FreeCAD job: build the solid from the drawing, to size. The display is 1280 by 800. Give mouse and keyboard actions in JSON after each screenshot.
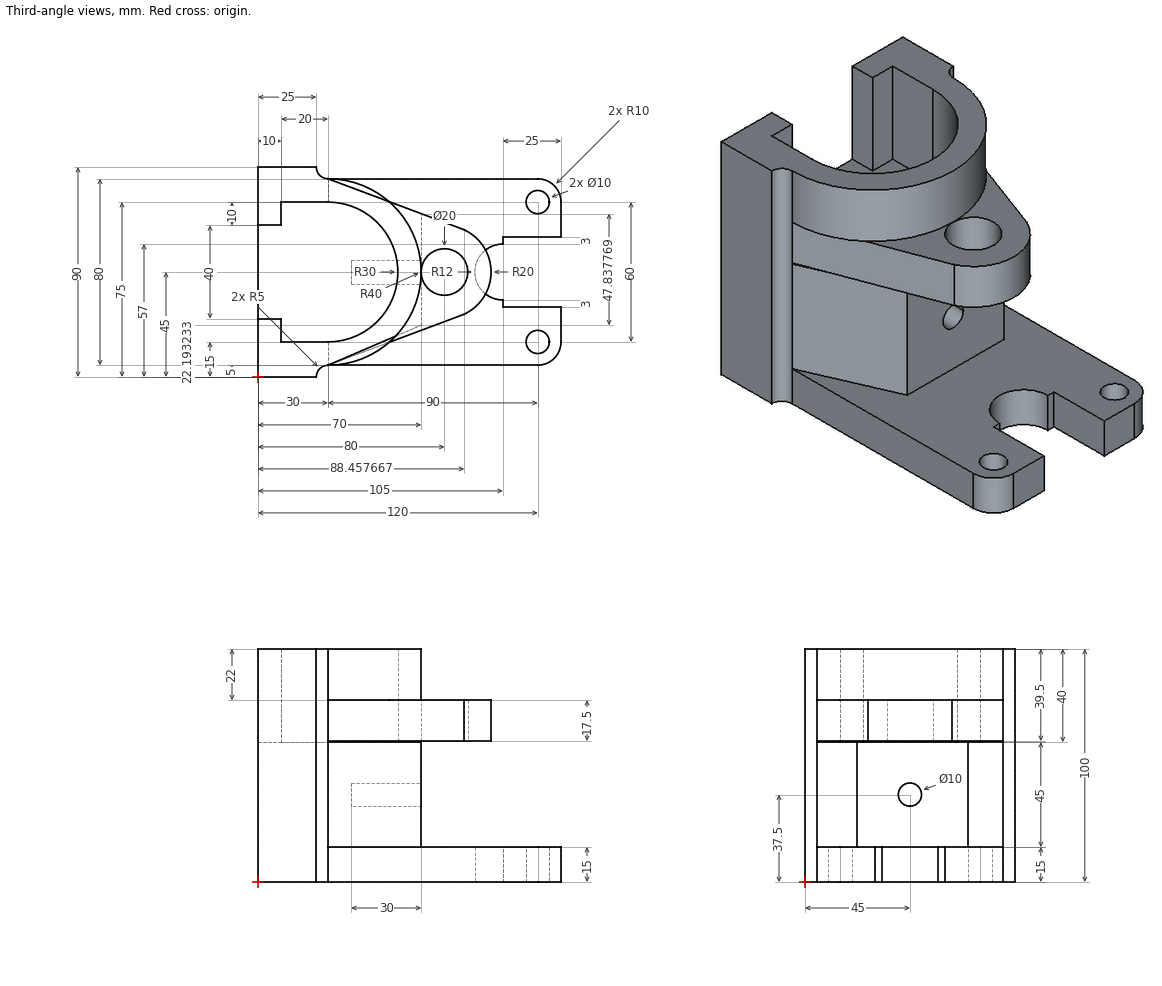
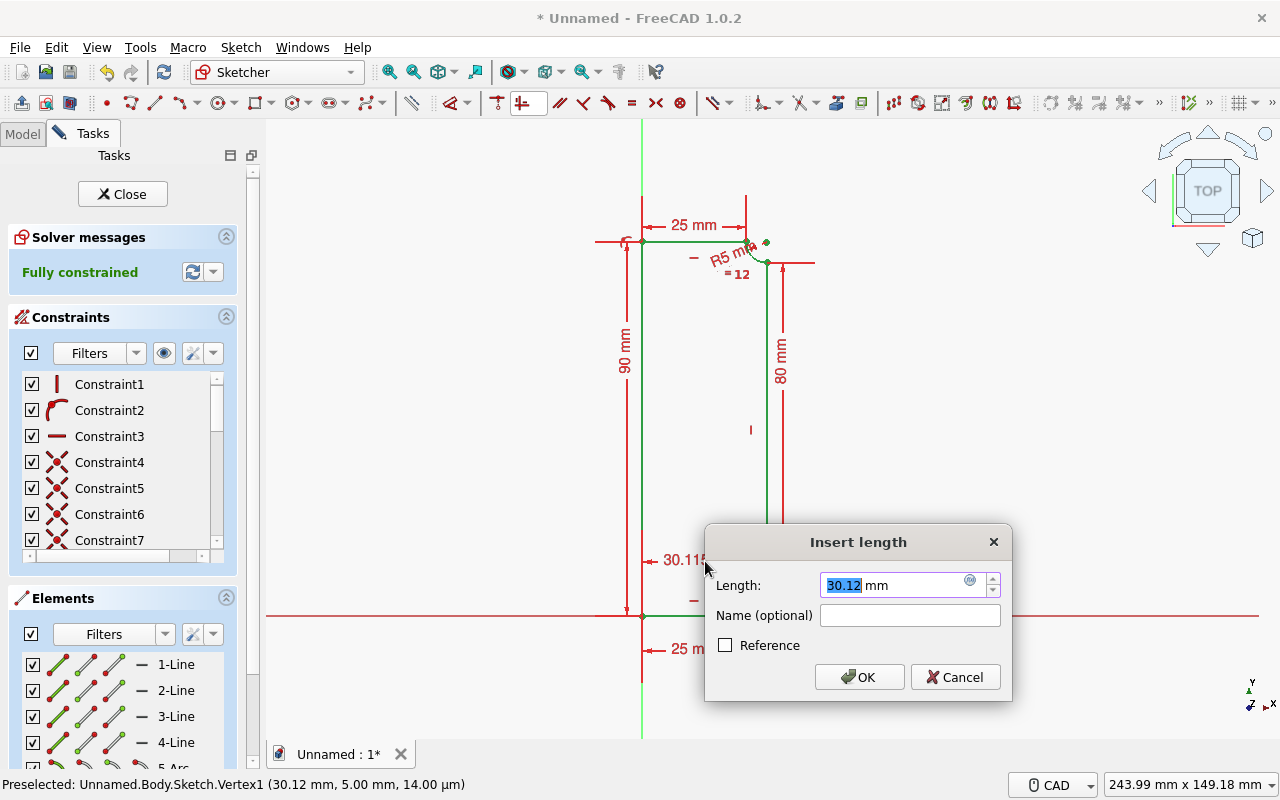
{"action": "type", "text": "30"}
{"action": "key", "text": "Return"}
{"action": "key", "text": "Escape"}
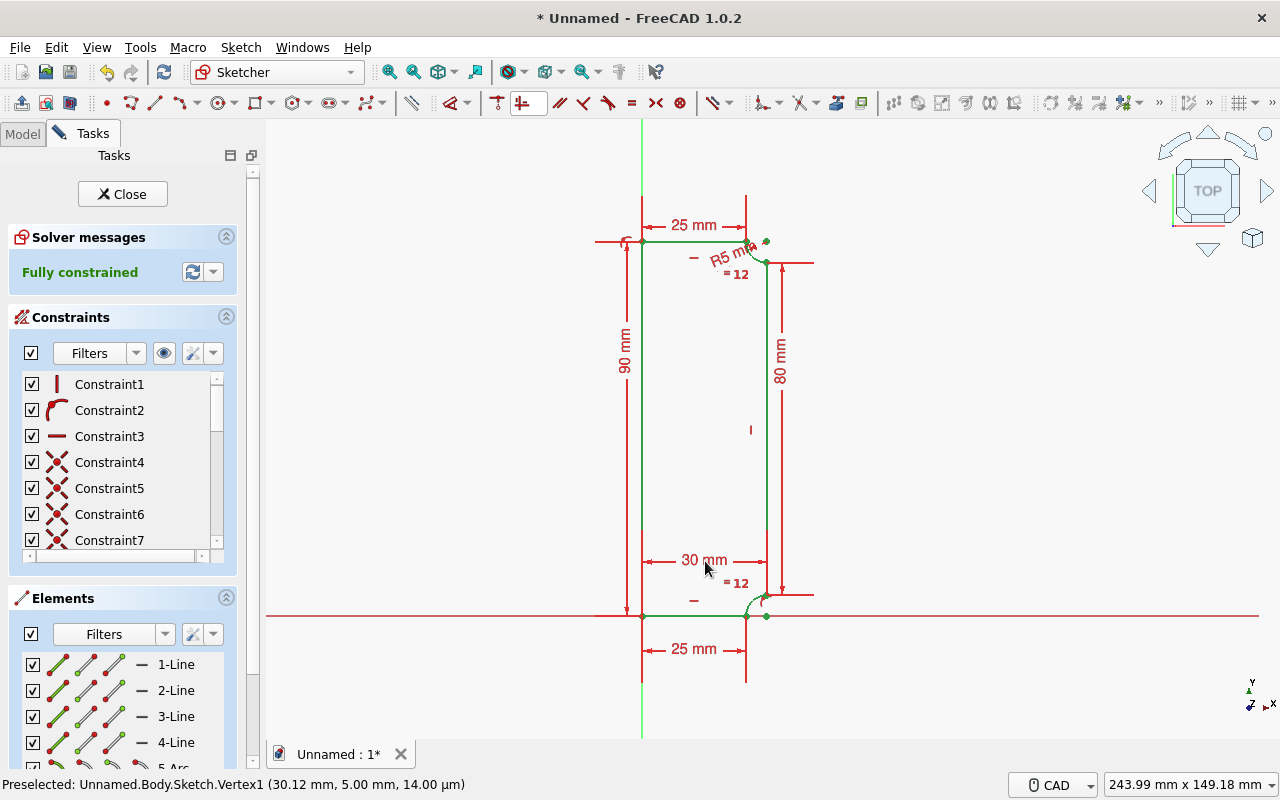
{"action": "left_click", "coordinate": [123, 194]}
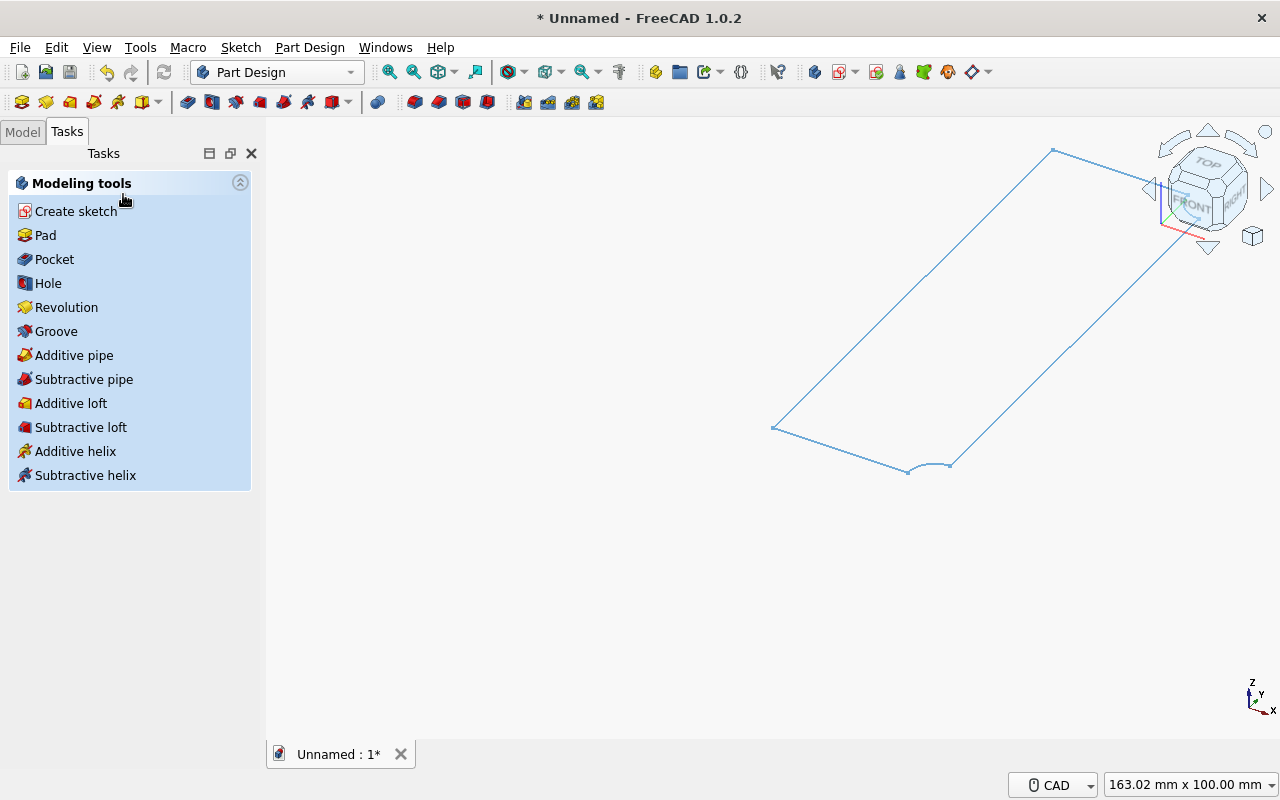
{"action": "left_click", "coordinate": [22, 102]}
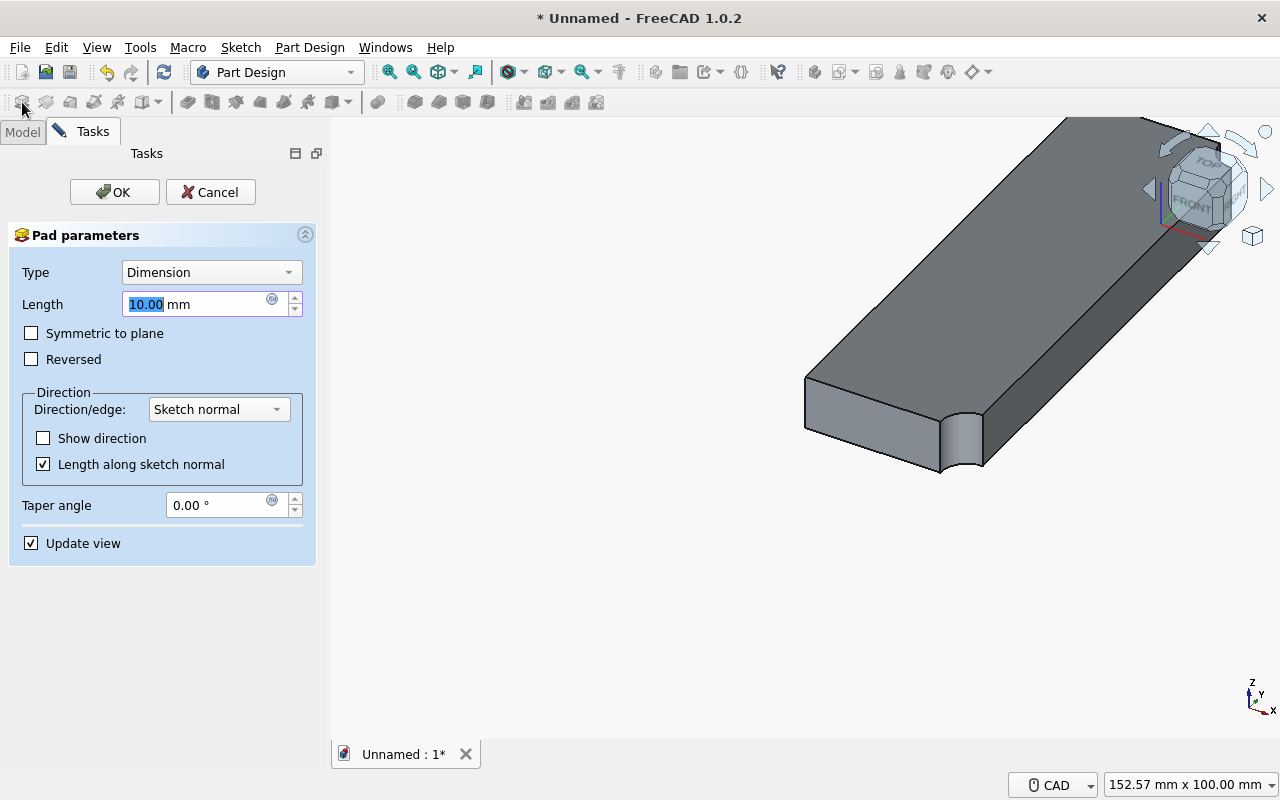
{"action": "type", "text": "100"}
{"action": "key", "text": "Tab"}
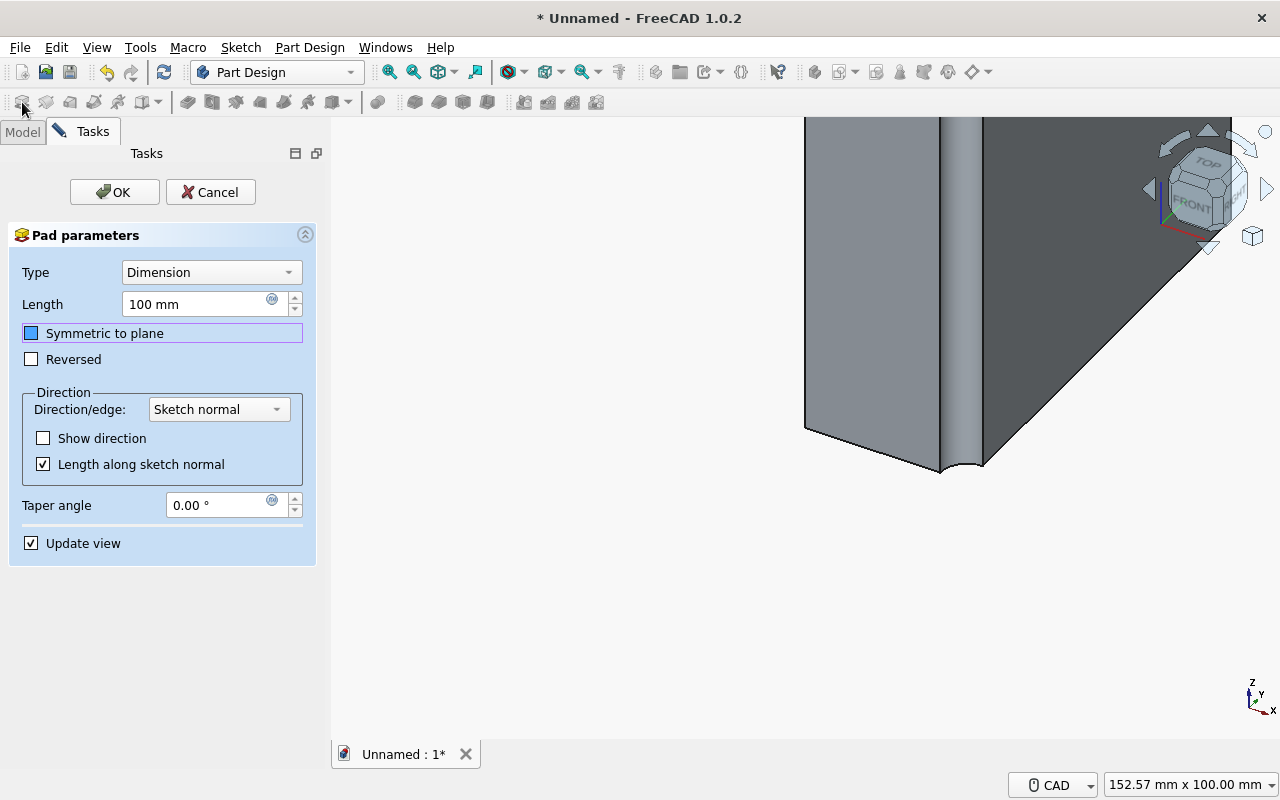
{"action": "left_click", "coordinate": [115, 192]}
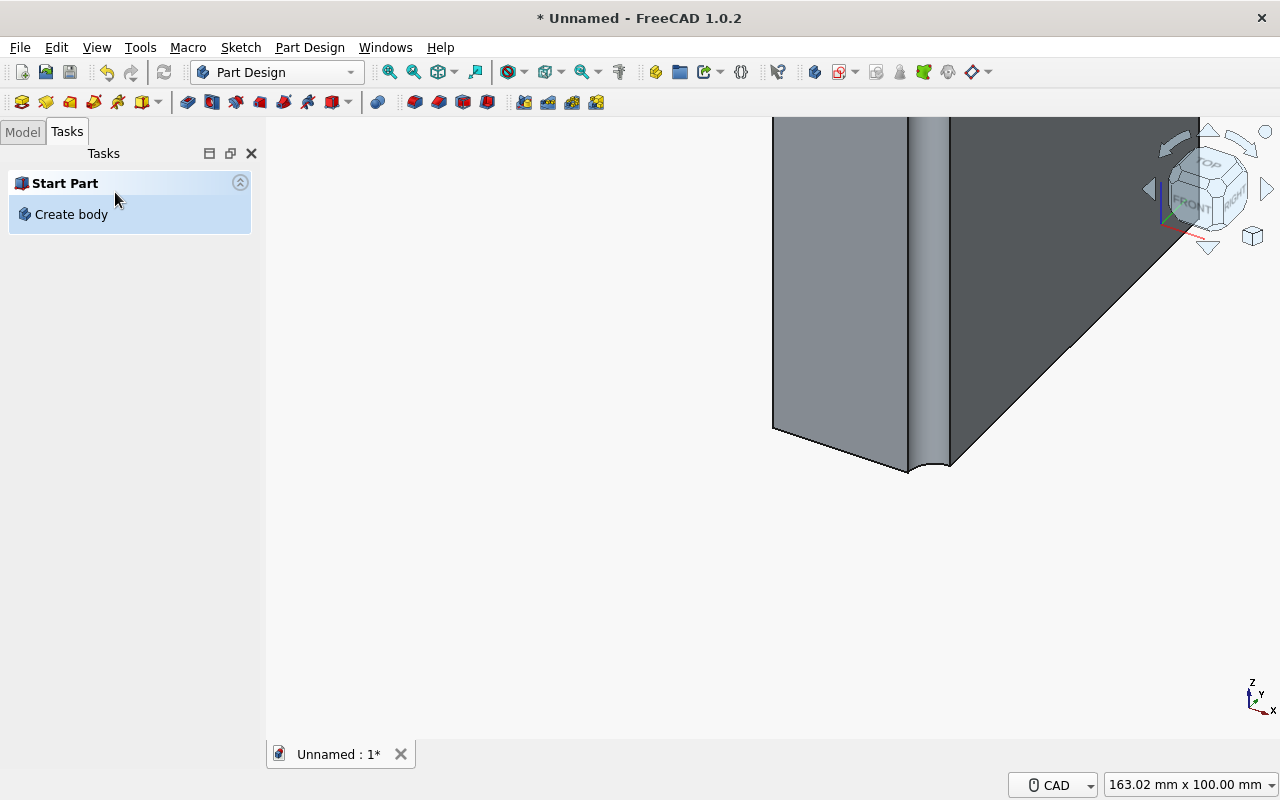
{"action": "left_click", "coordinate": [390, 72]}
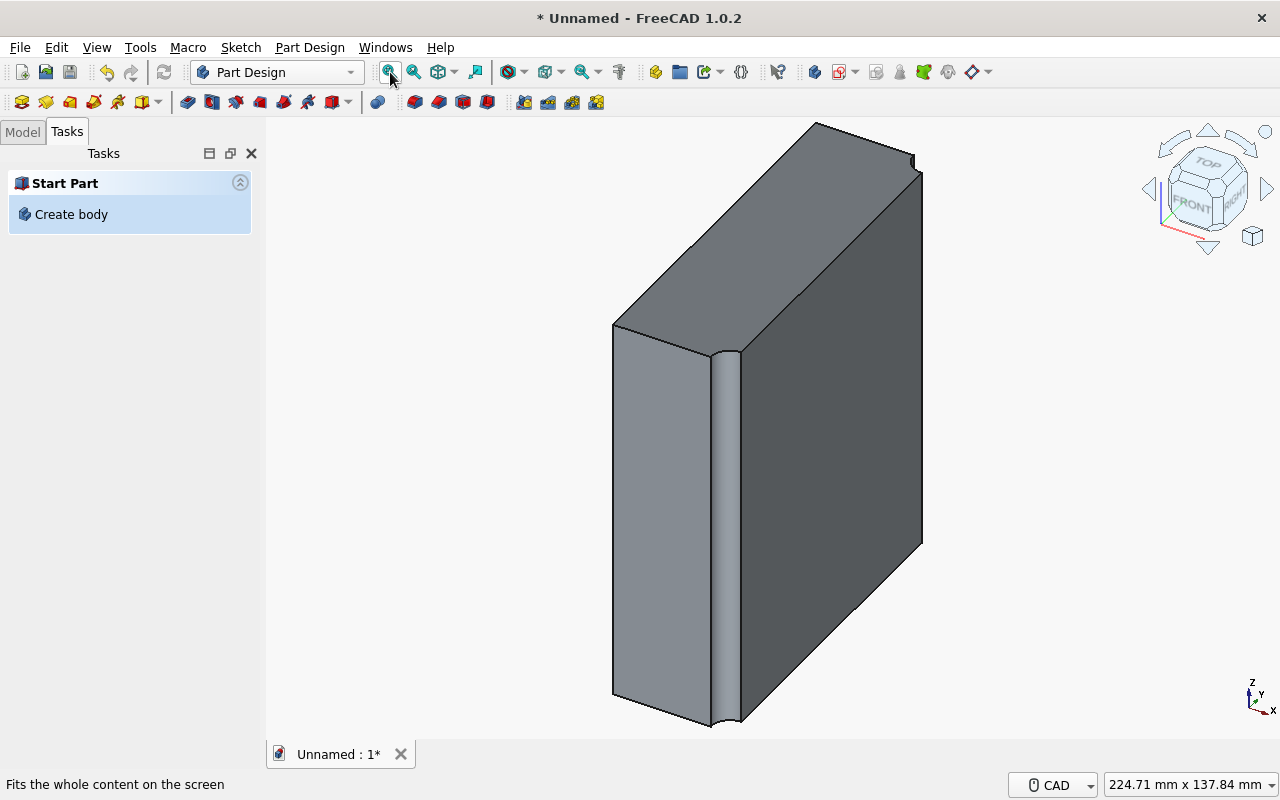
{"action": "left_click", "coordinate": [840, 72]}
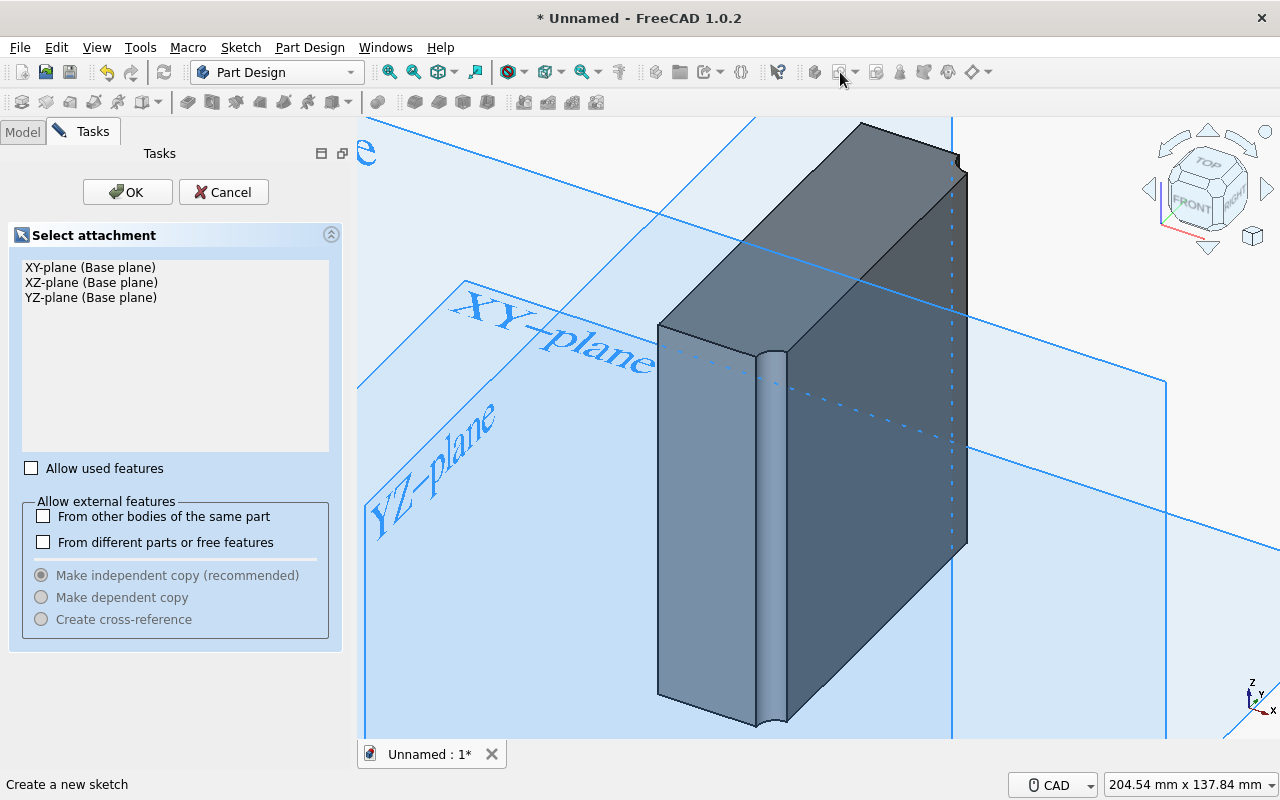
{"action": "left_click", "coordinate": [82, 268]}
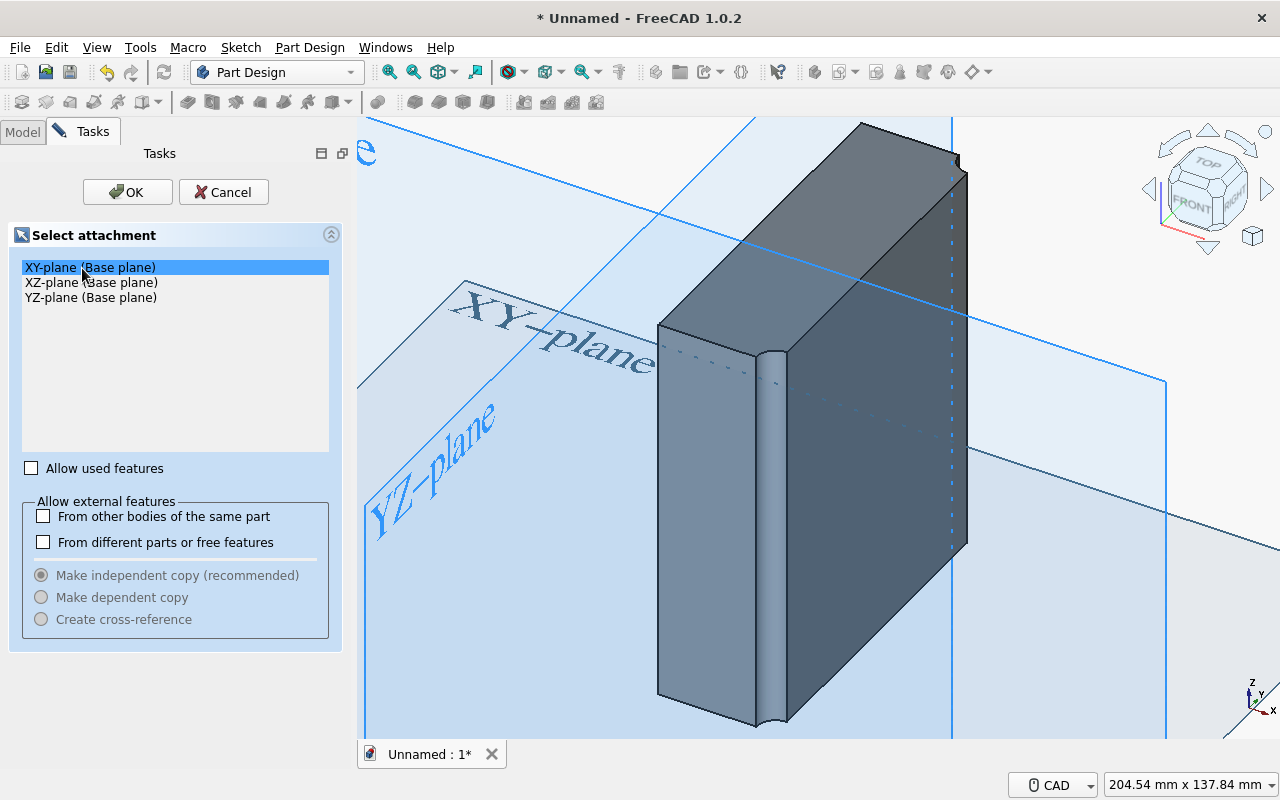
{"action": "left_click", "coordinate": [128, 192]}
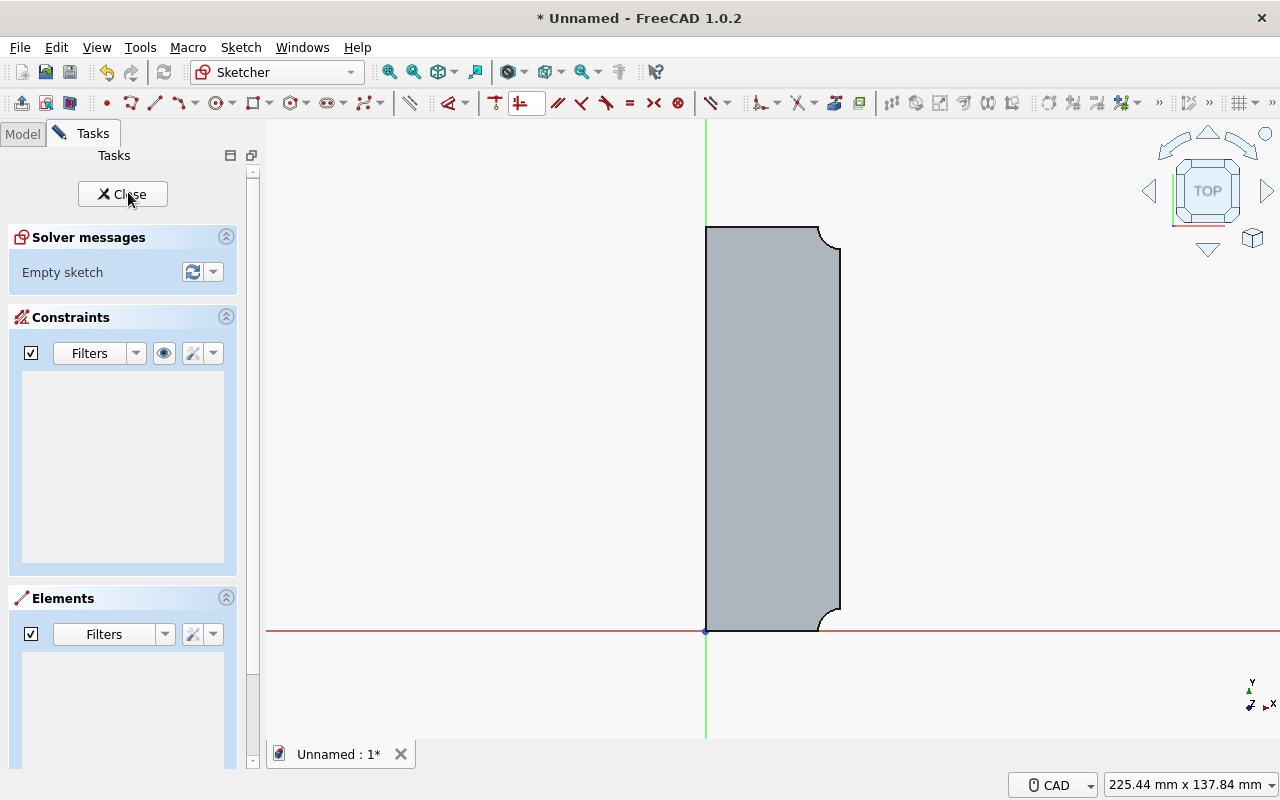
{"action": "left_click", "coordinate": [70, 104]}